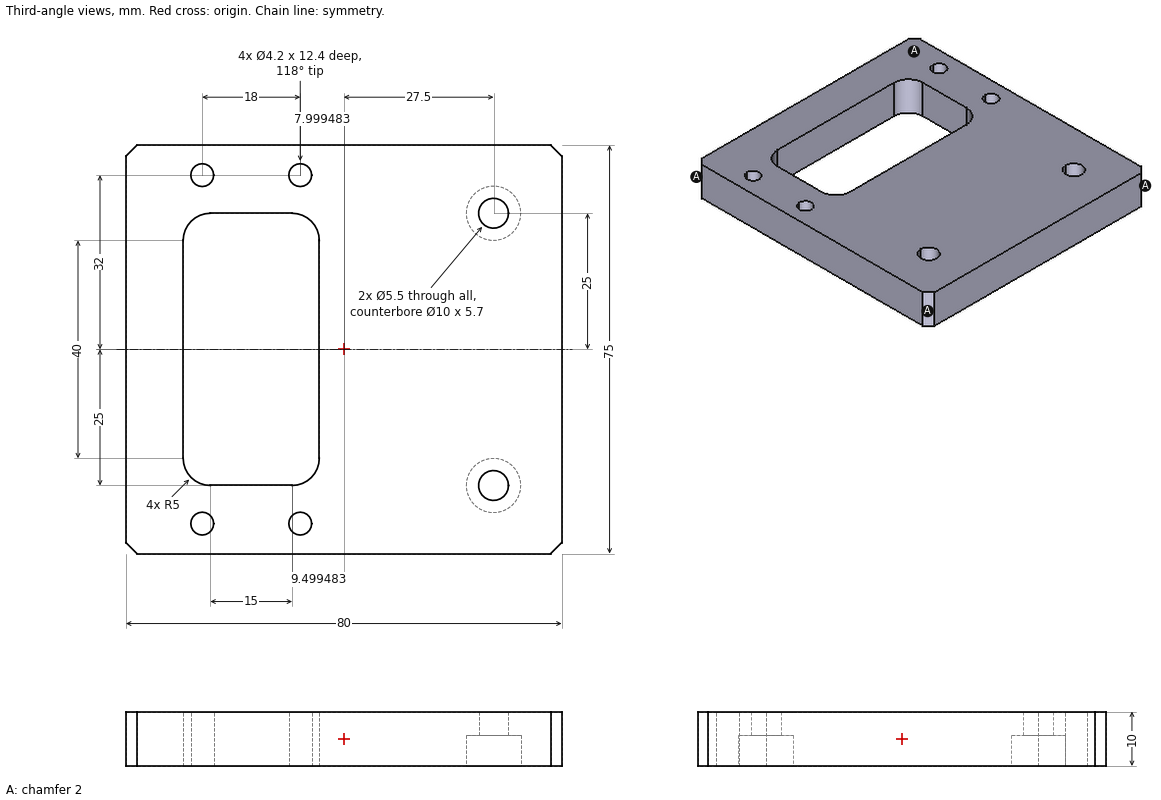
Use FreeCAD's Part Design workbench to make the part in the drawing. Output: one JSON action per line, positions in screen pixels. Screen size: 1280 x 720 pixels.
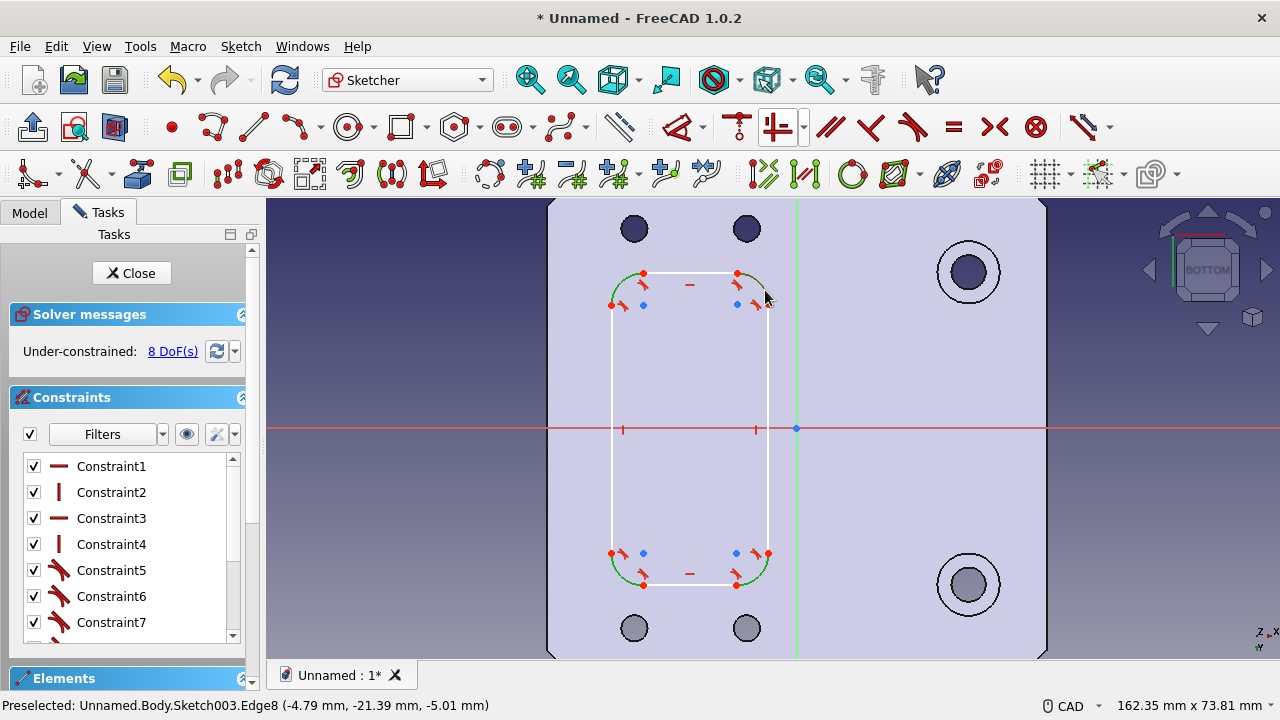
{"action": "left_click", "coordinate": [954, 128]}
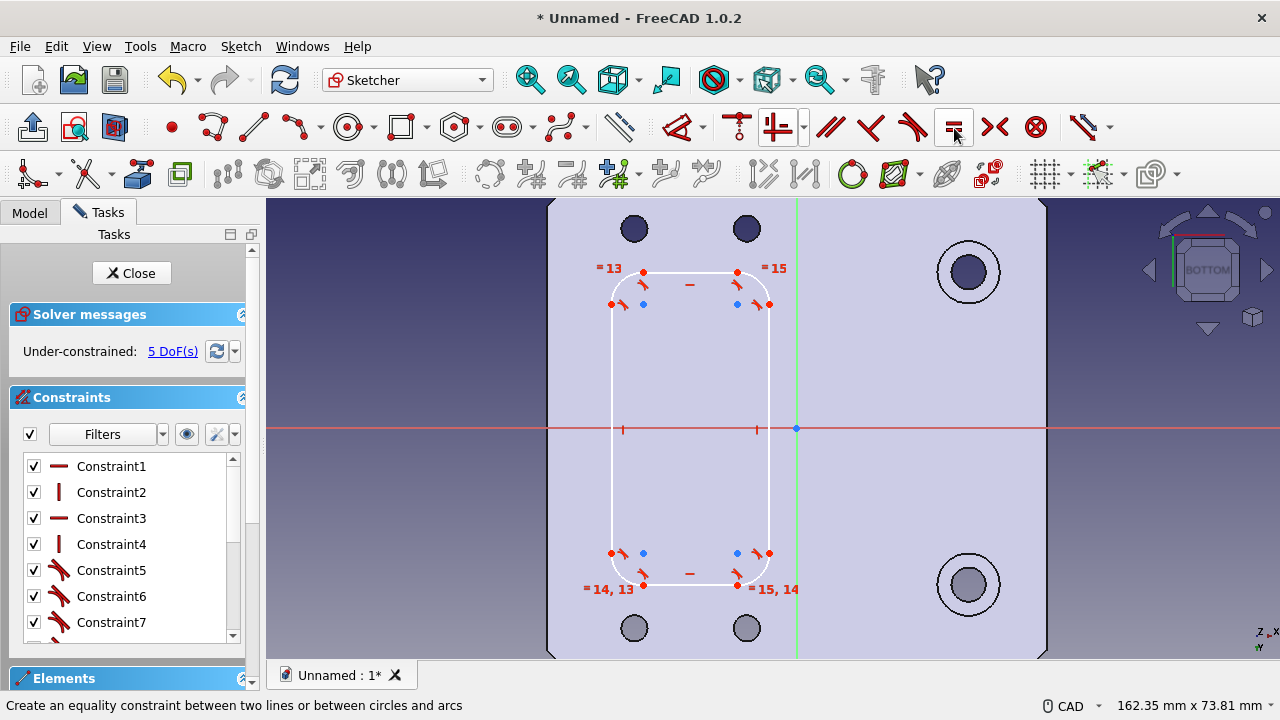
{"action": "left_click", "coordinate": [676, 128]}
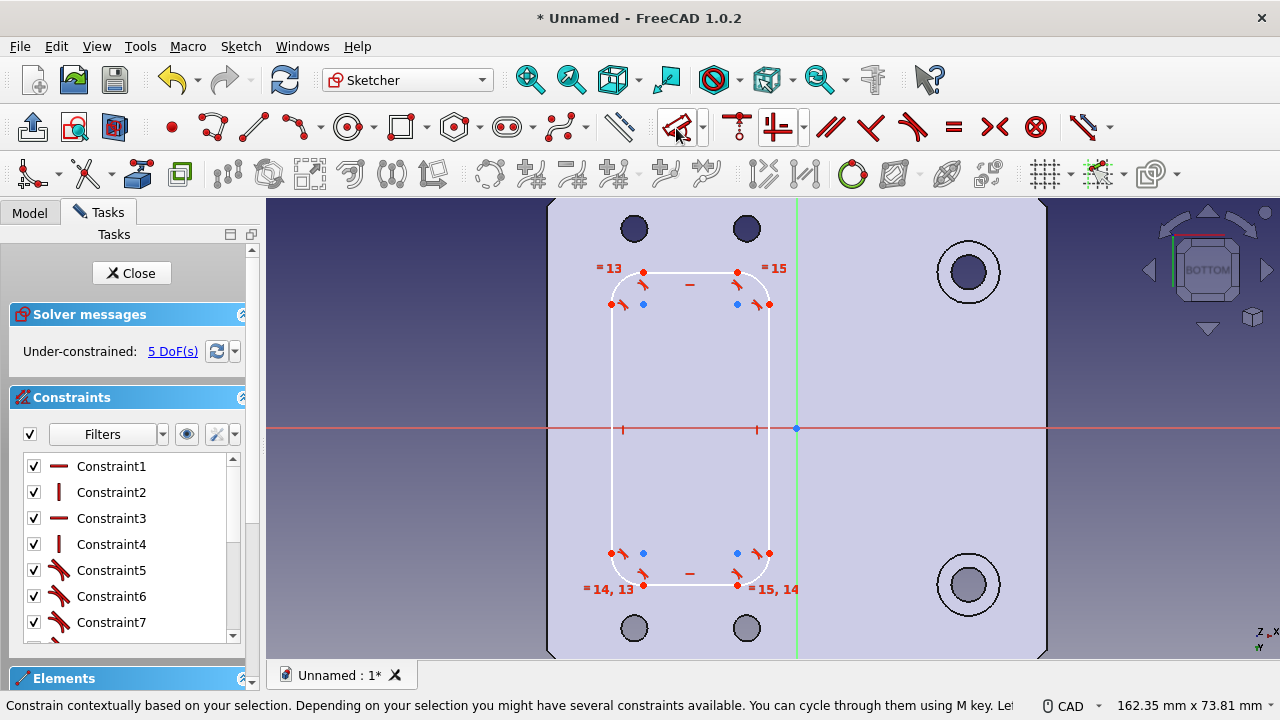
{"action": "scroll", "coordinate": [629, 276], "scroll_direction": "up", "scroll_amount": 2}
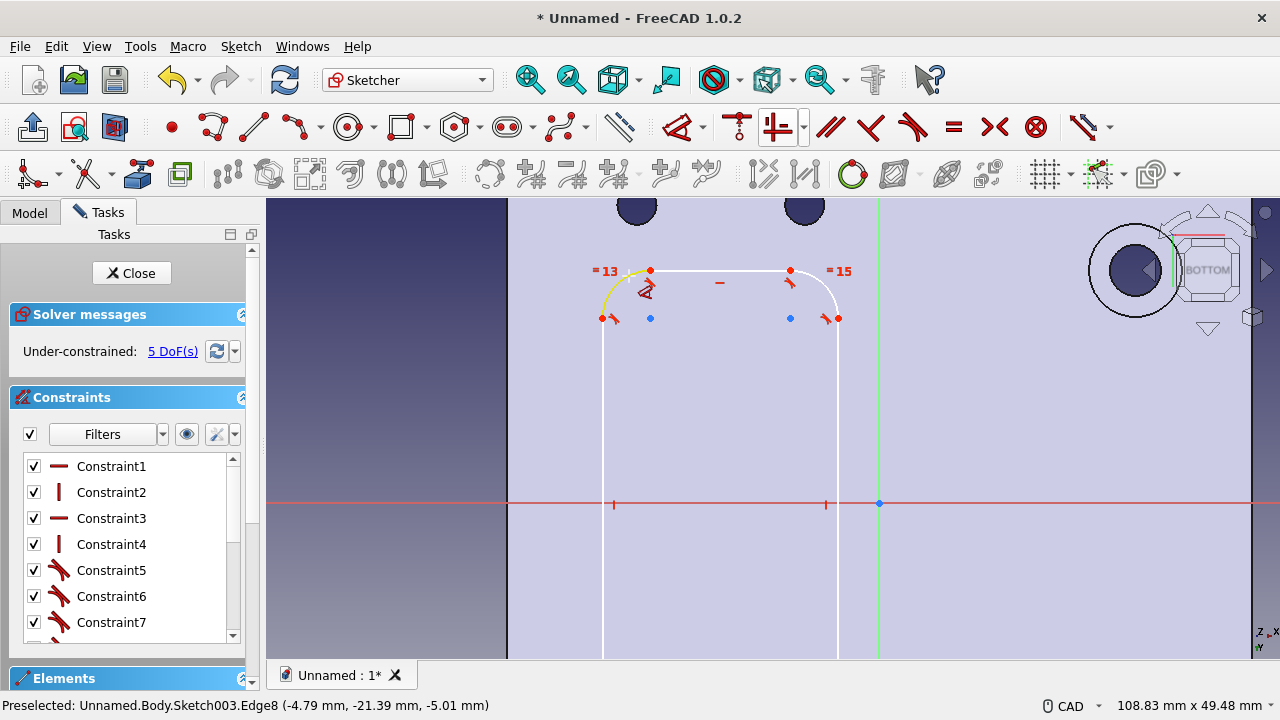
{"action": "left_click", "coordinate": [629, 276]}
{"action": "left_click", "coordinate": [615, 247]}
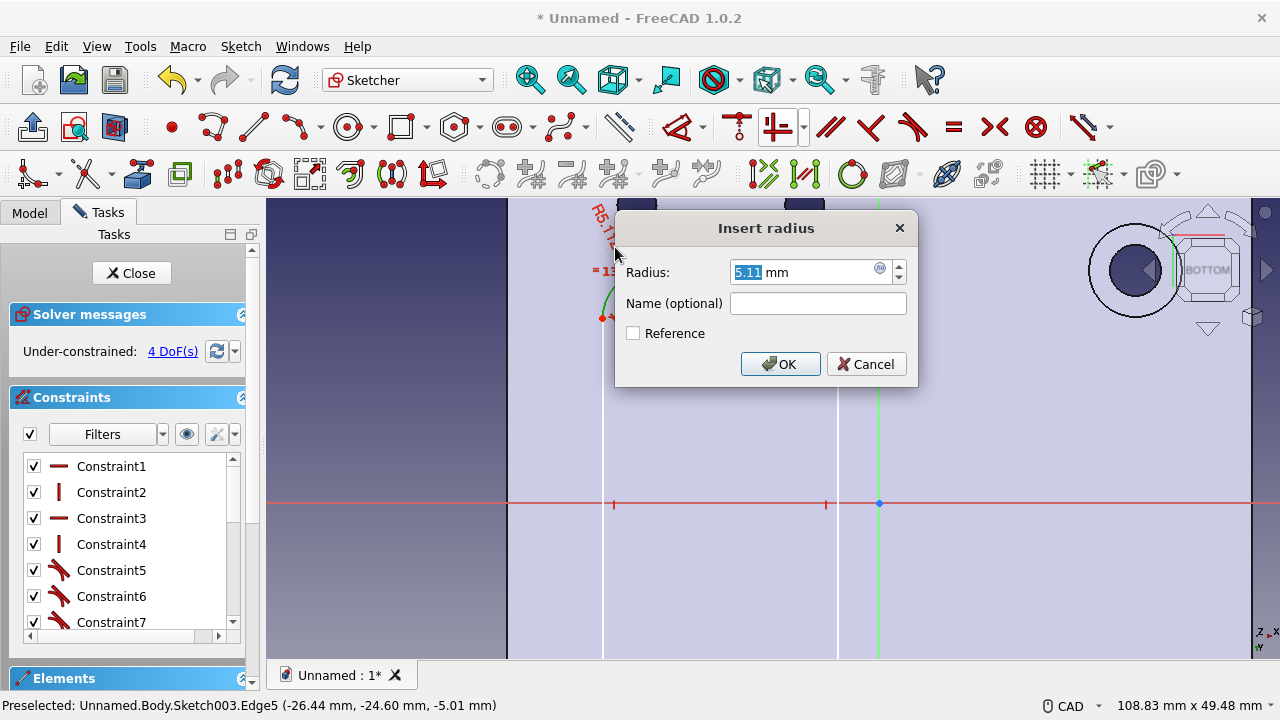
{"action": "type", "text": "5"}
{"action": "key", "text": "Return"}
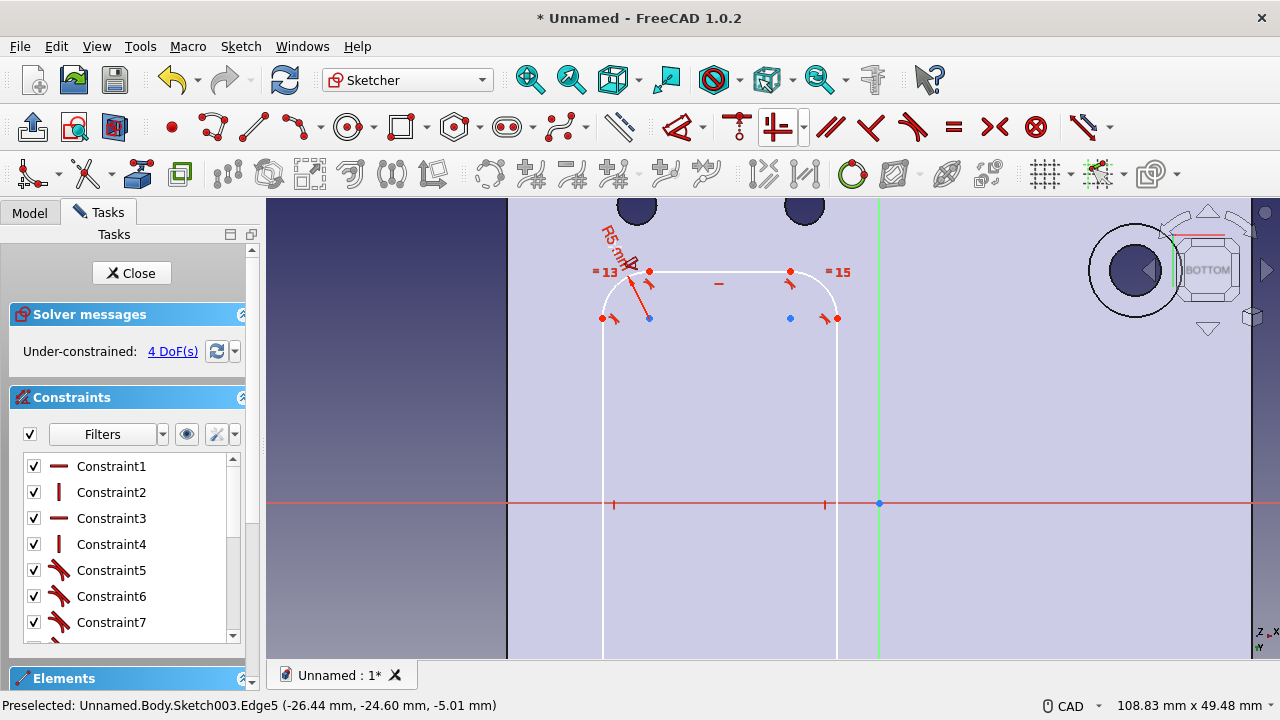
{"action": "left_click", "coordinate": [748, 272]}
{"action": "left_click", "coordinate": [720, 238]}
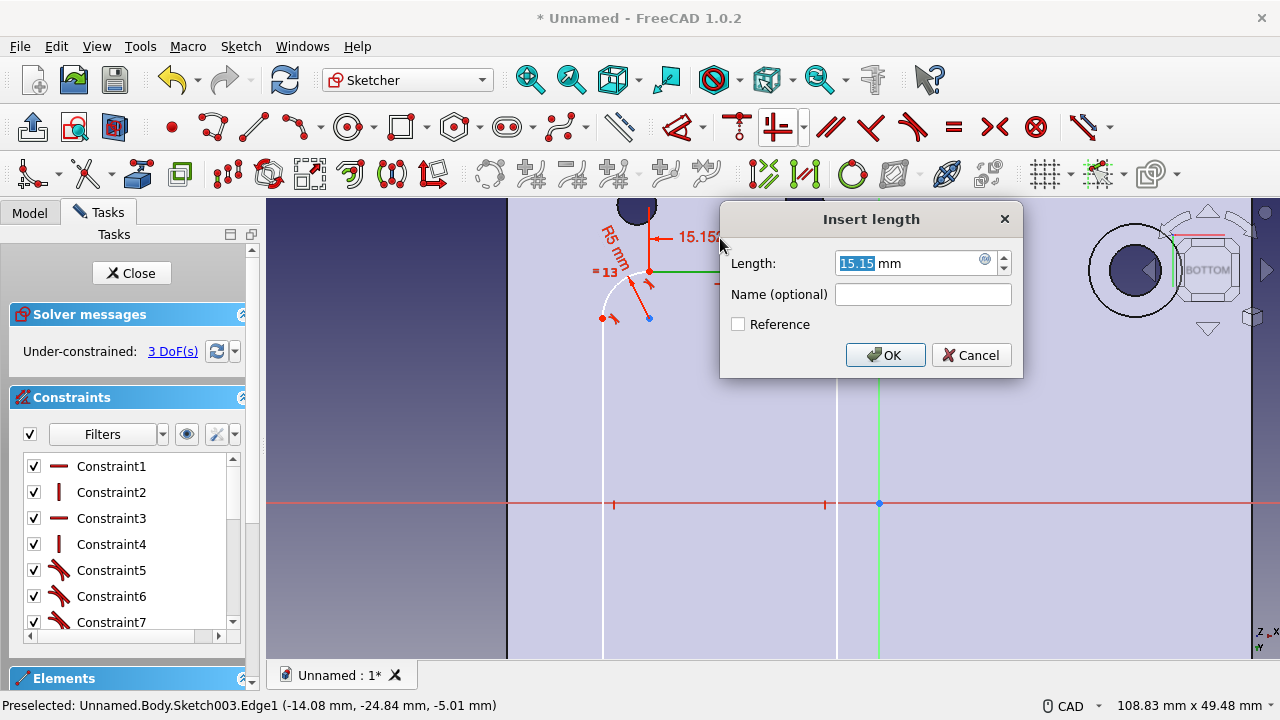
{"action": "type", "text": "15"}
{"action": "key", "text": "Return"}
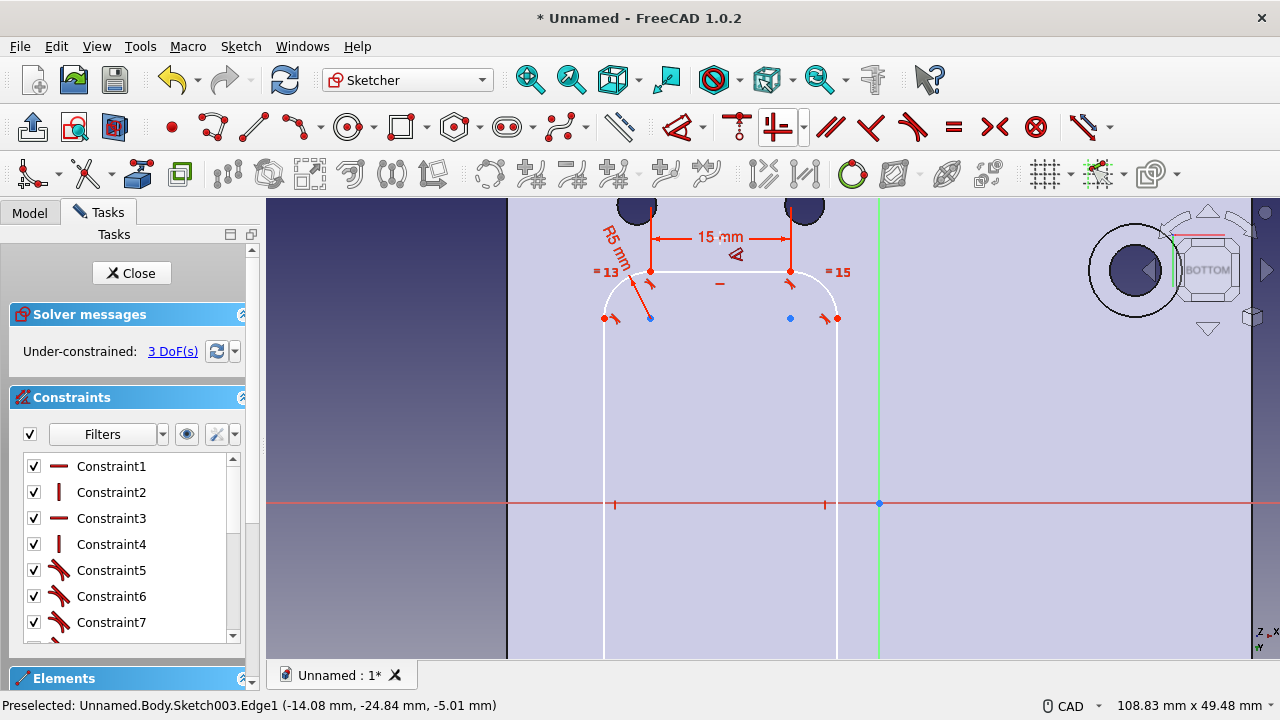
{"action": "left_click", "coordinate": [604, 430]}
{"action": "left_click", "coordinate": [570, 475]}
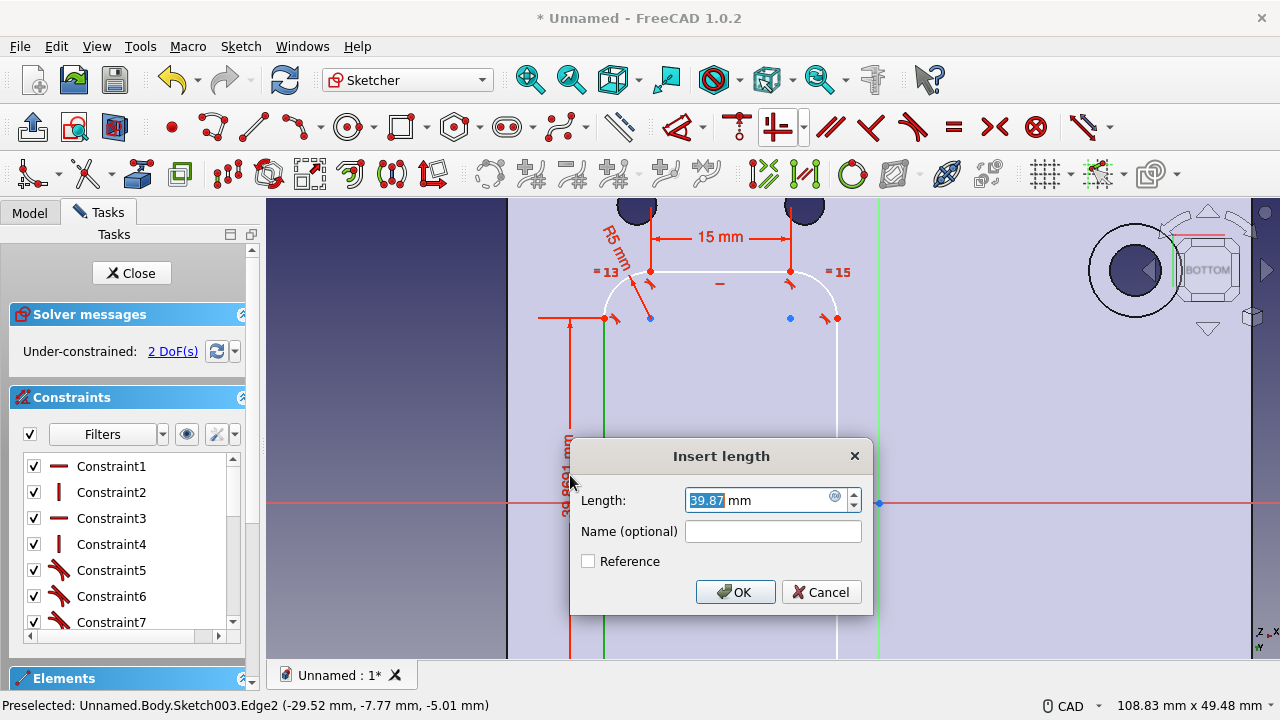
{"action": "type", "text": "40"}
{"action": "key", "text": "Return"}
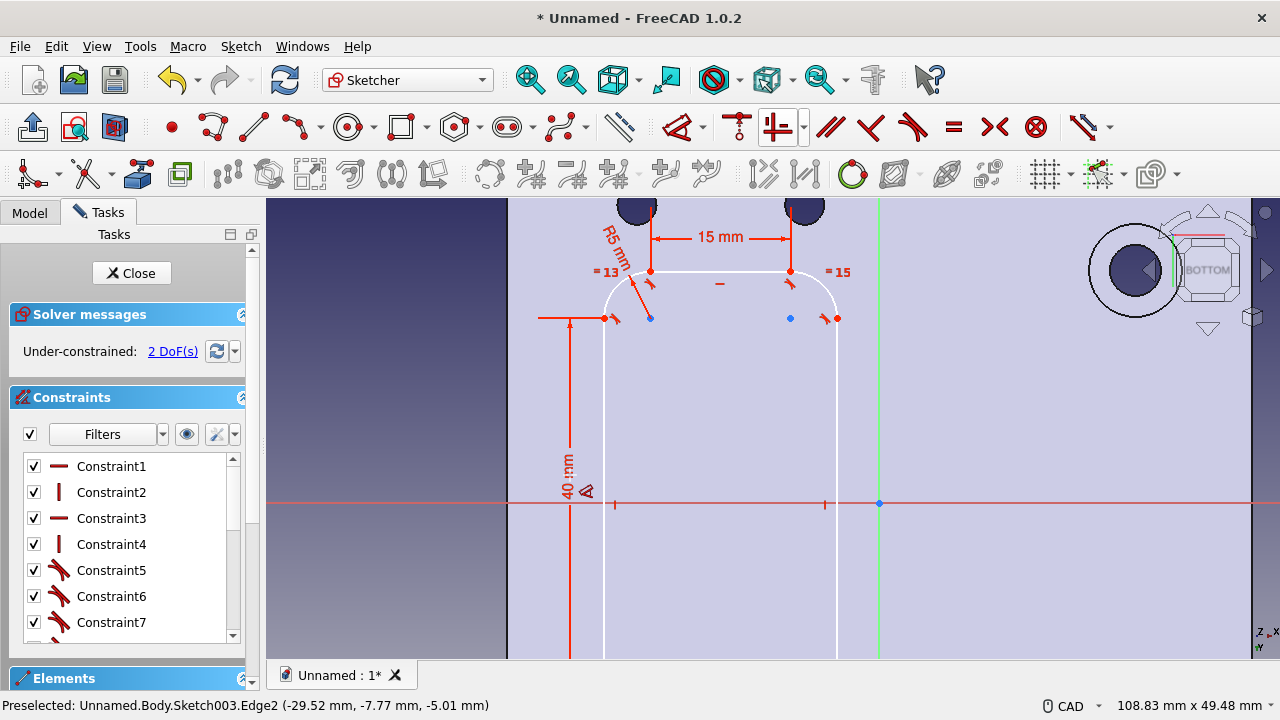
{"action": "left_click", "coordinate": [791, 272]}
{"action": "left_click", "coordinate": [913, 388]}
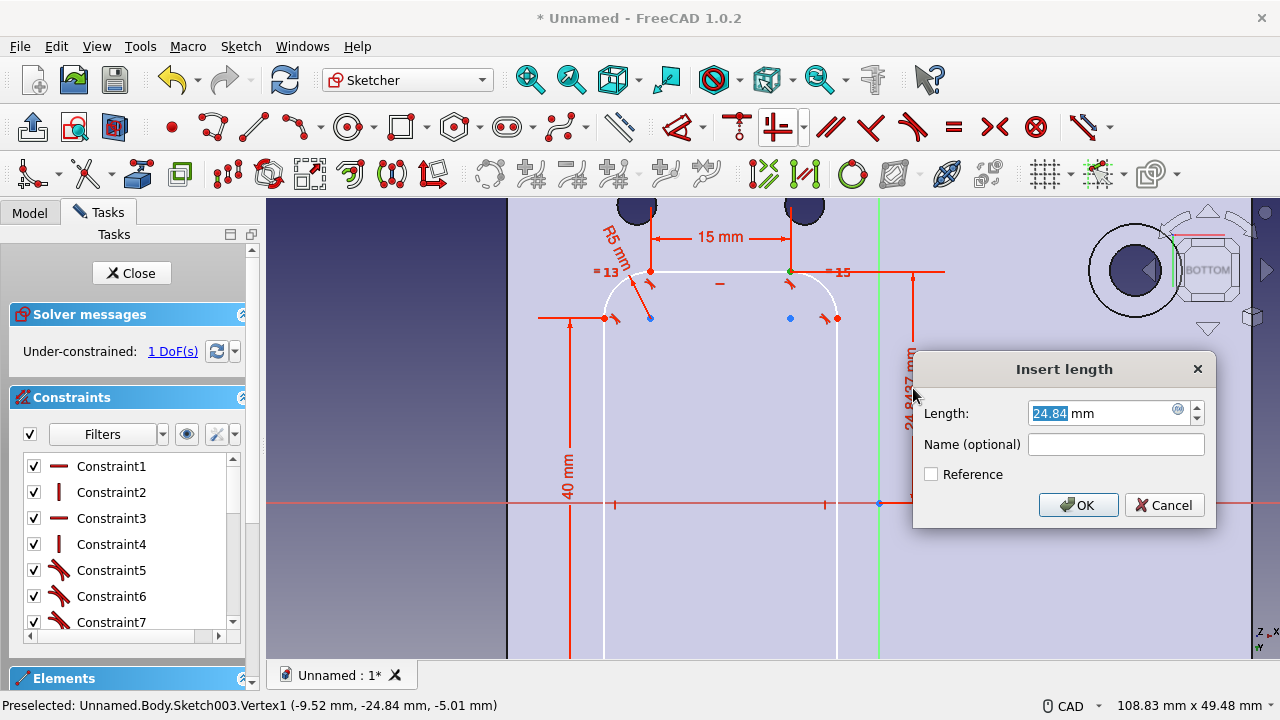
{"action": "type", "text": "25"}
{"action": "key", "text": "Return"}